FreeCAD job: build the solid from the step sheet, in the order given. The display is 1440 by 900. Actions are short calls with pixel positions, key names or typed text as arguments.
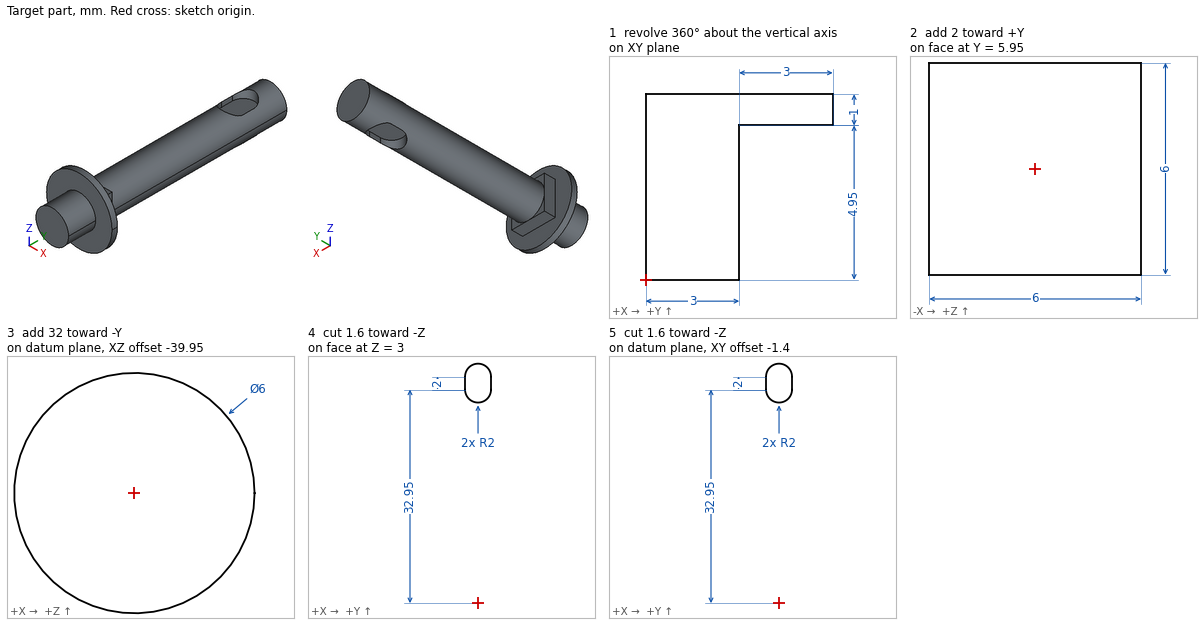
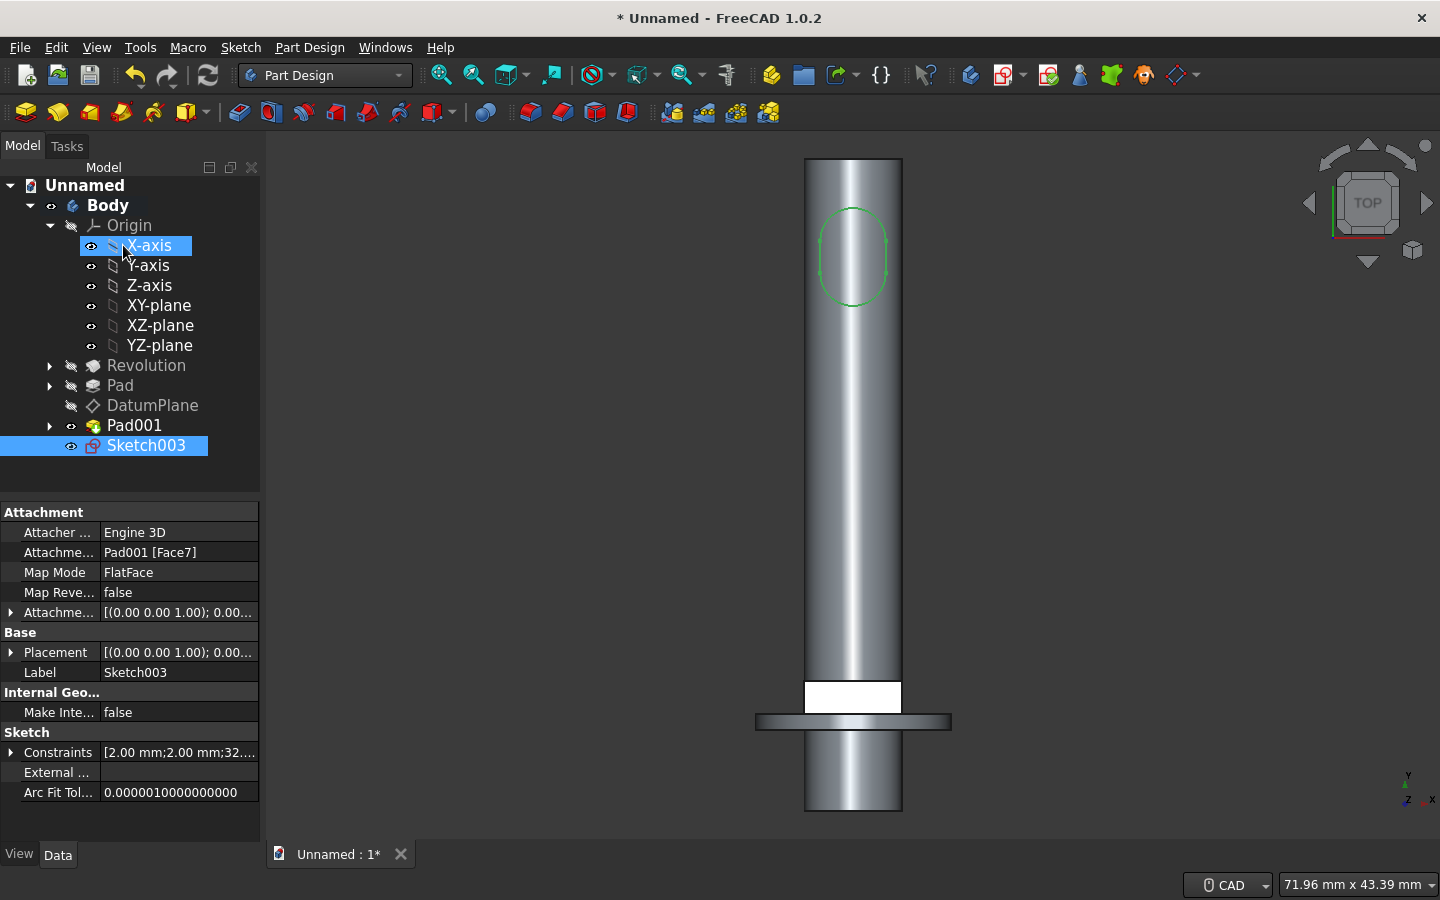
click(240, 112)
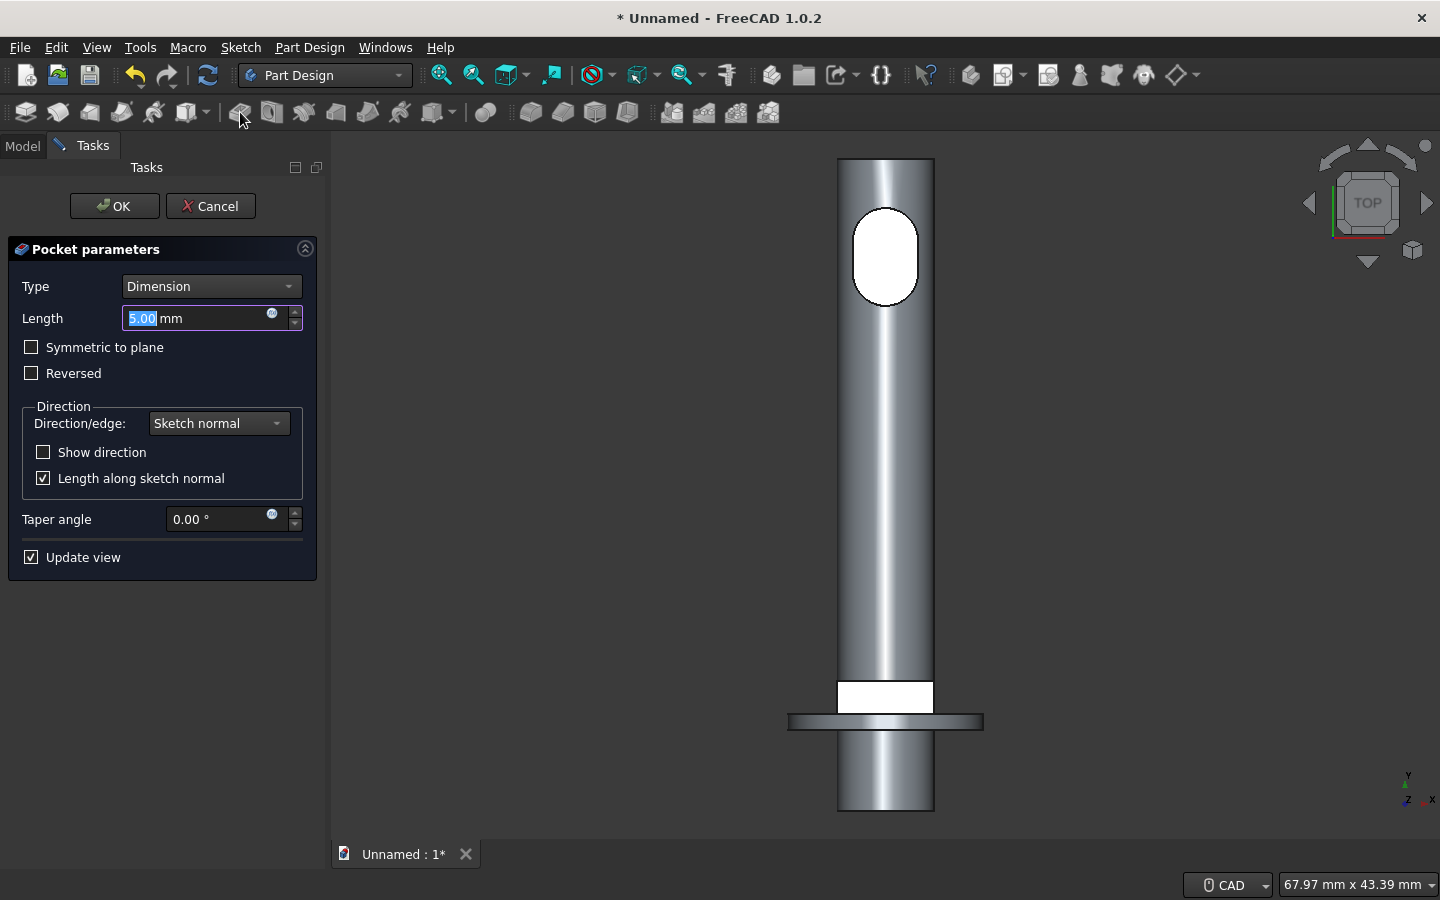
text(1.6)
key(Tab)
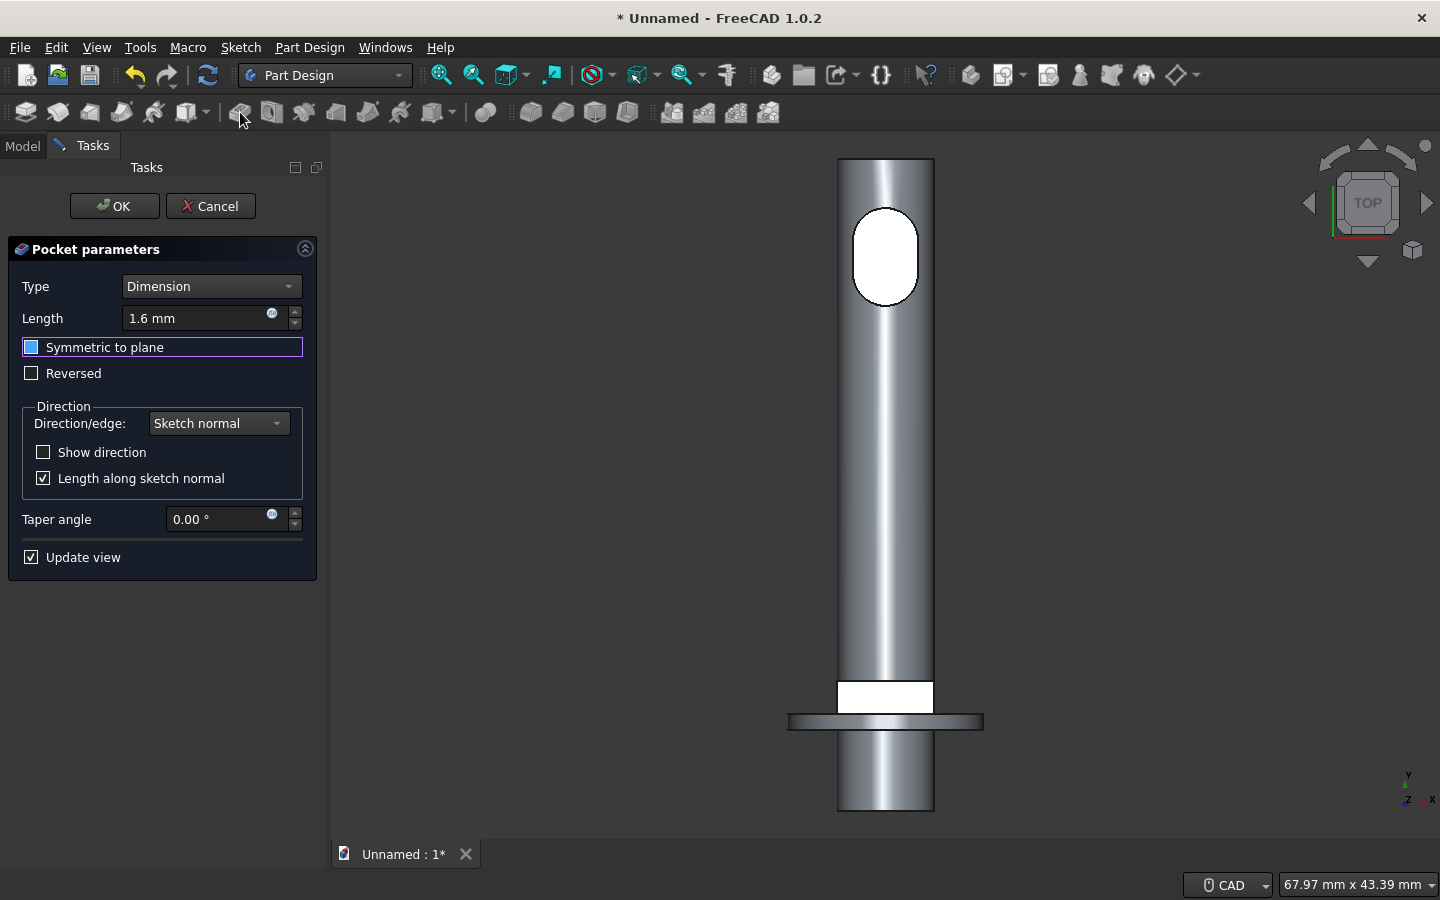
click(115, 206)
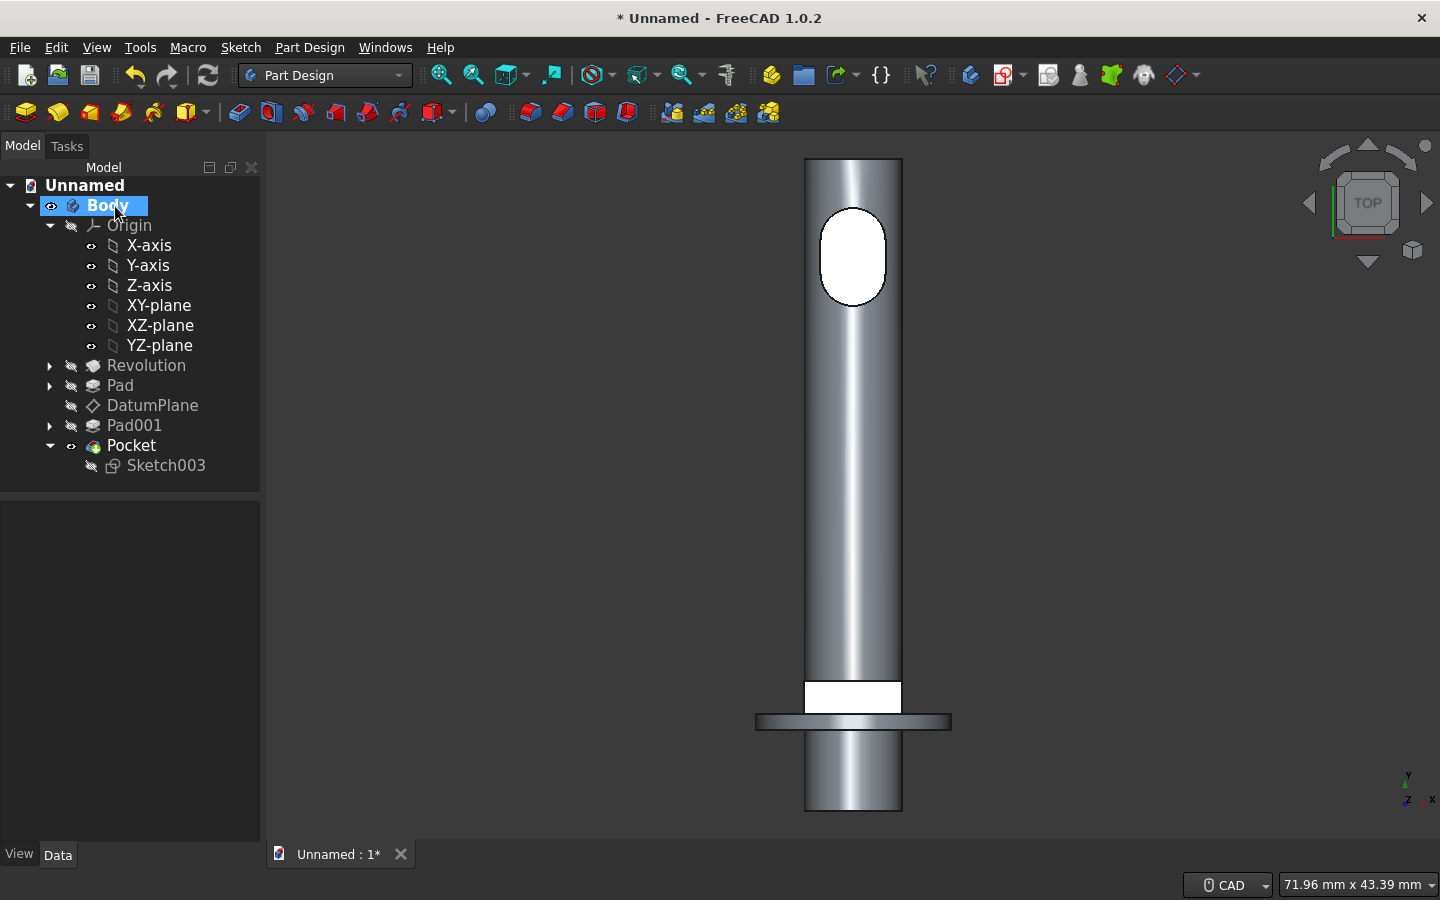
click(136, 306)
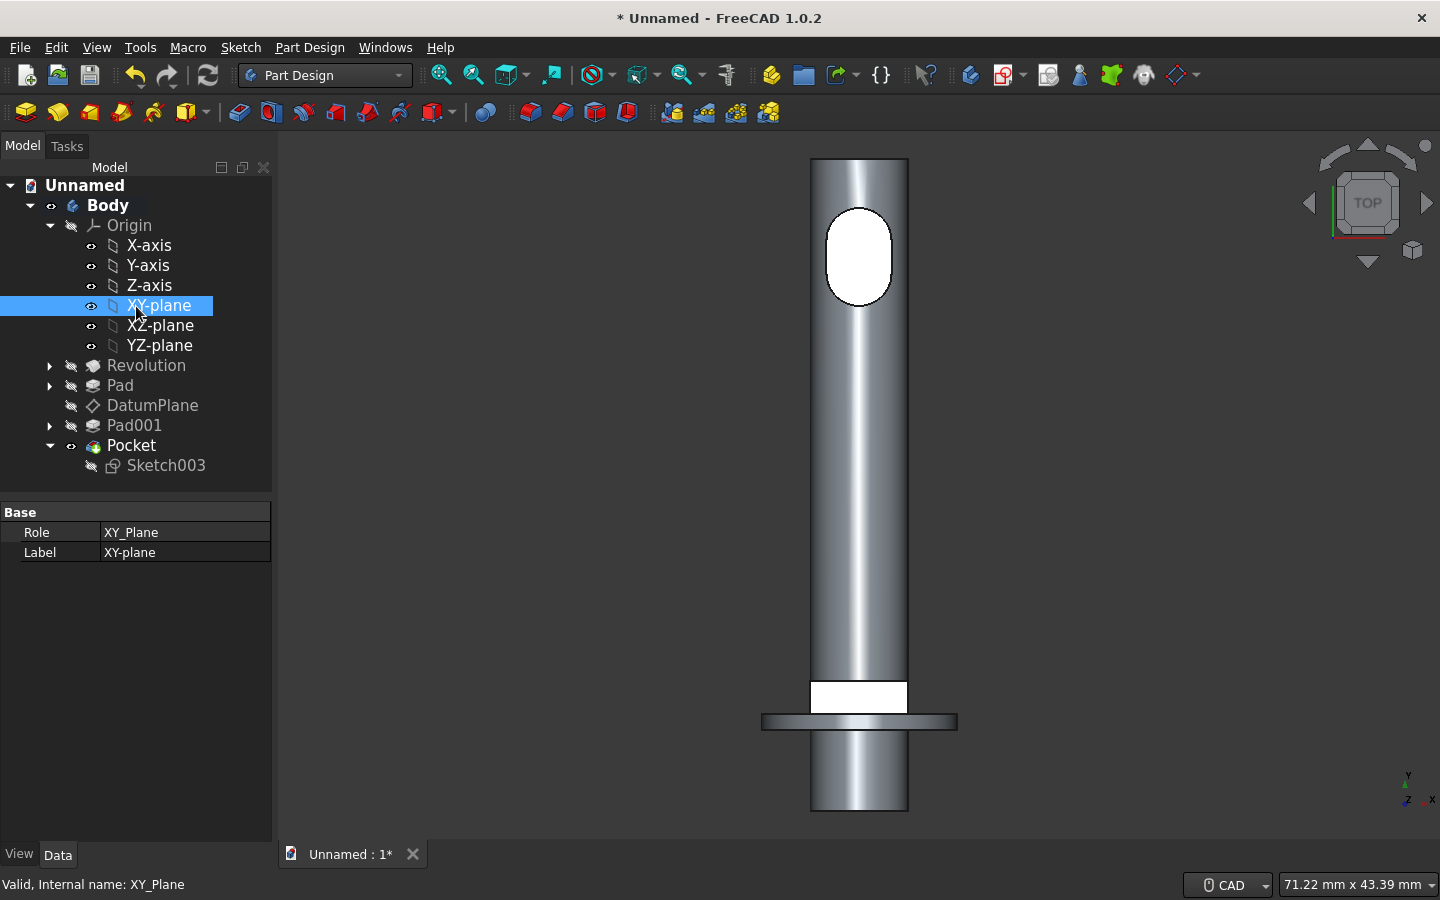
click(1176, 76)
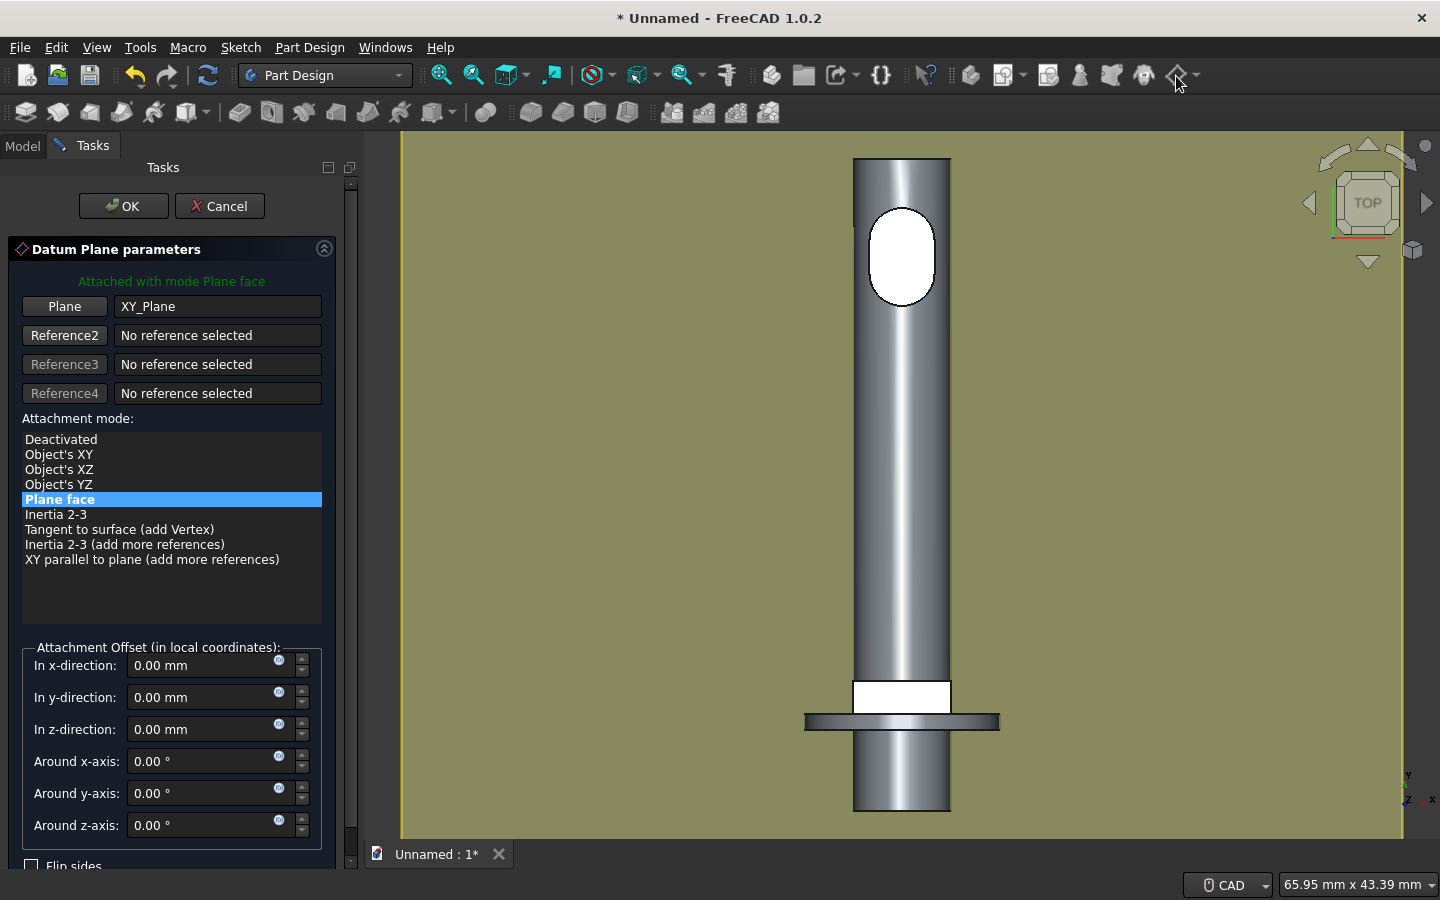
triple_click(210, 729)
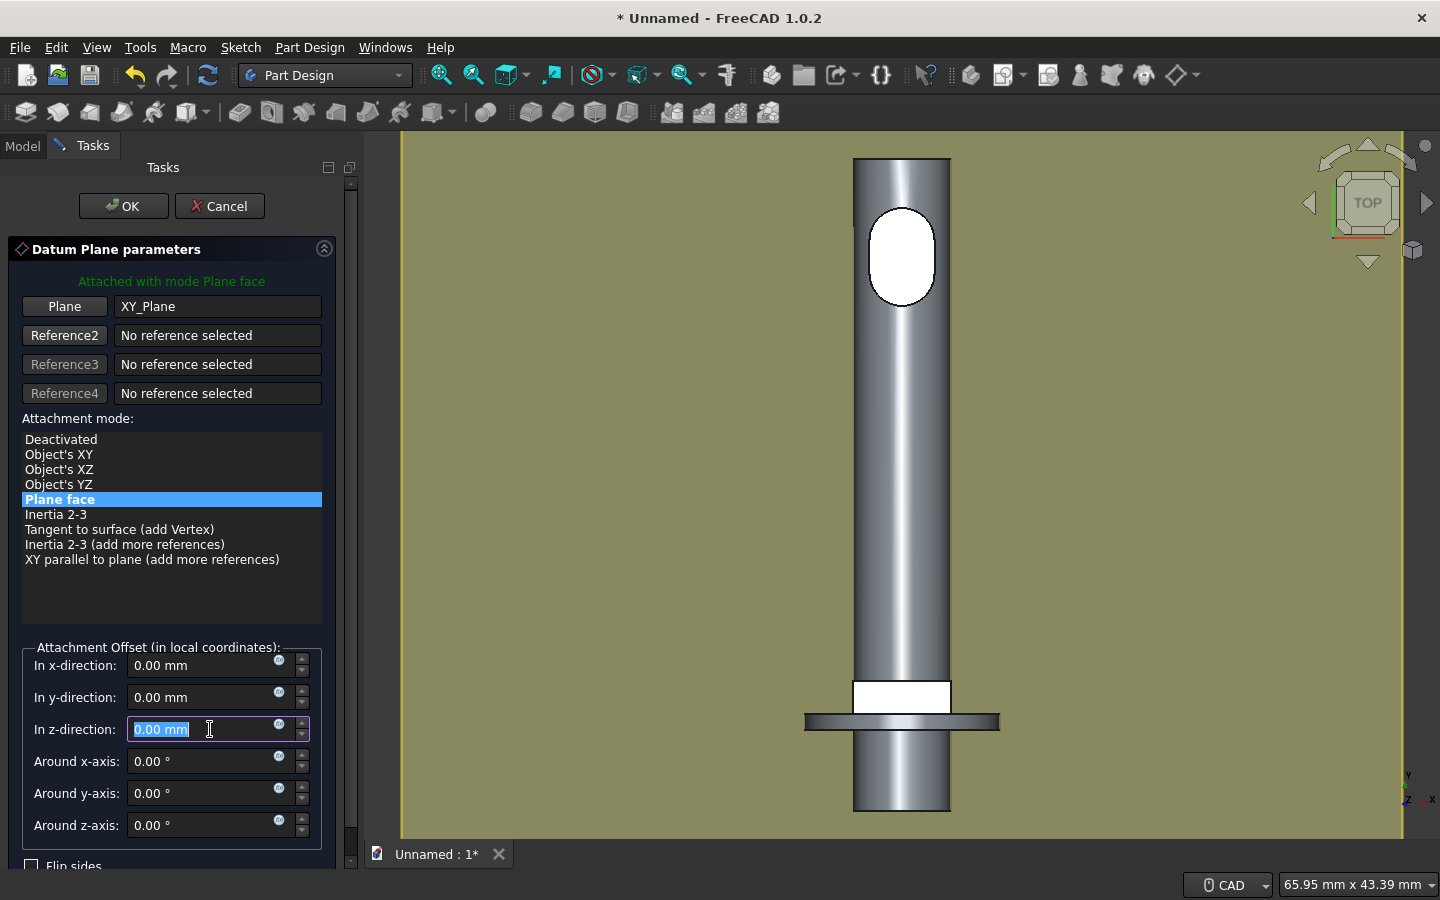
text(-1.4)
key(Tab)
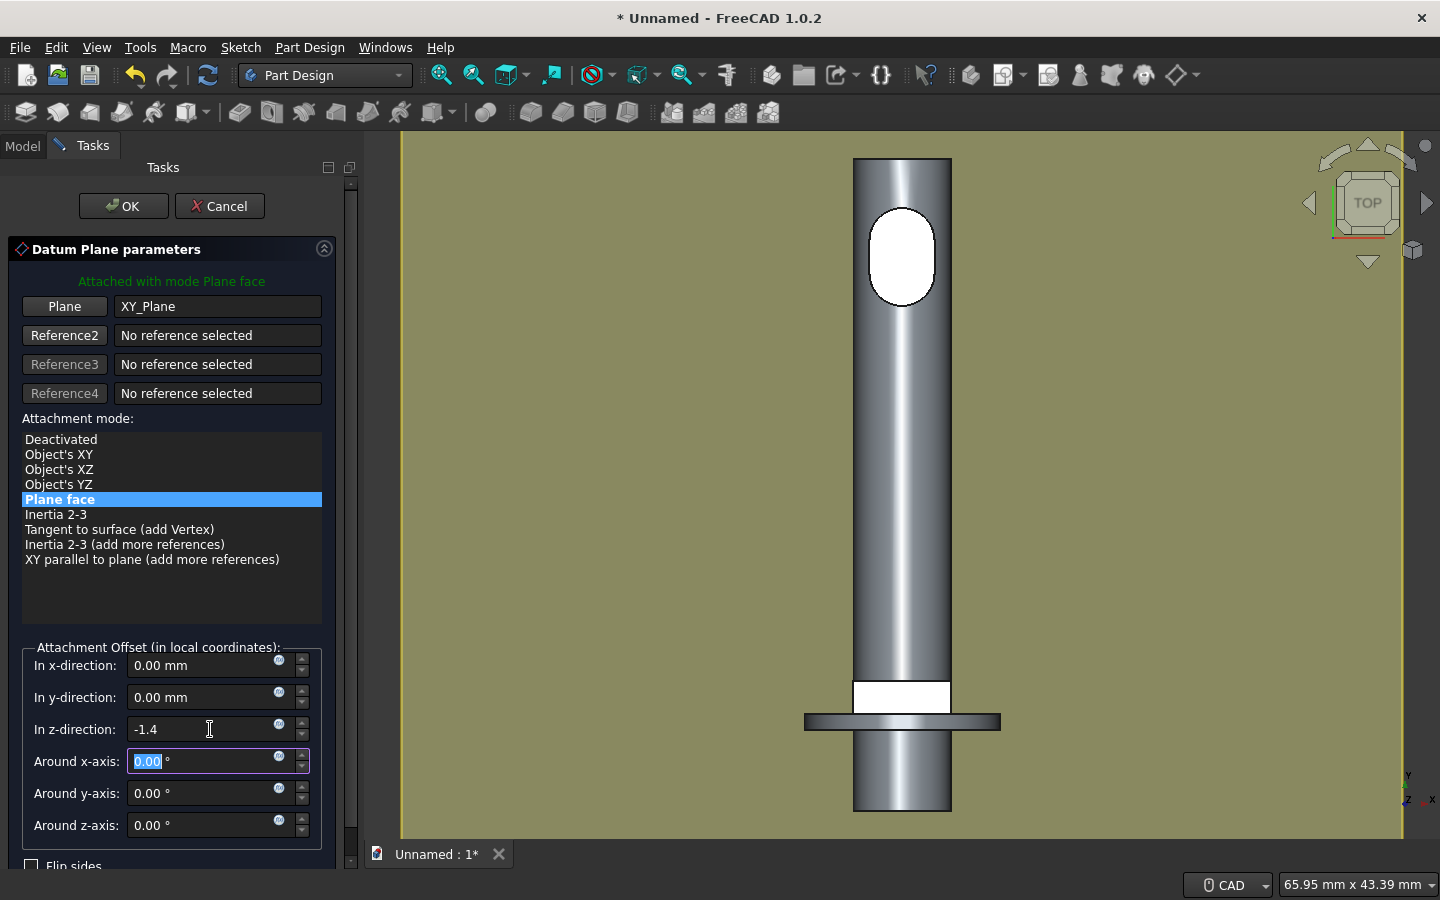
click(124, 206)